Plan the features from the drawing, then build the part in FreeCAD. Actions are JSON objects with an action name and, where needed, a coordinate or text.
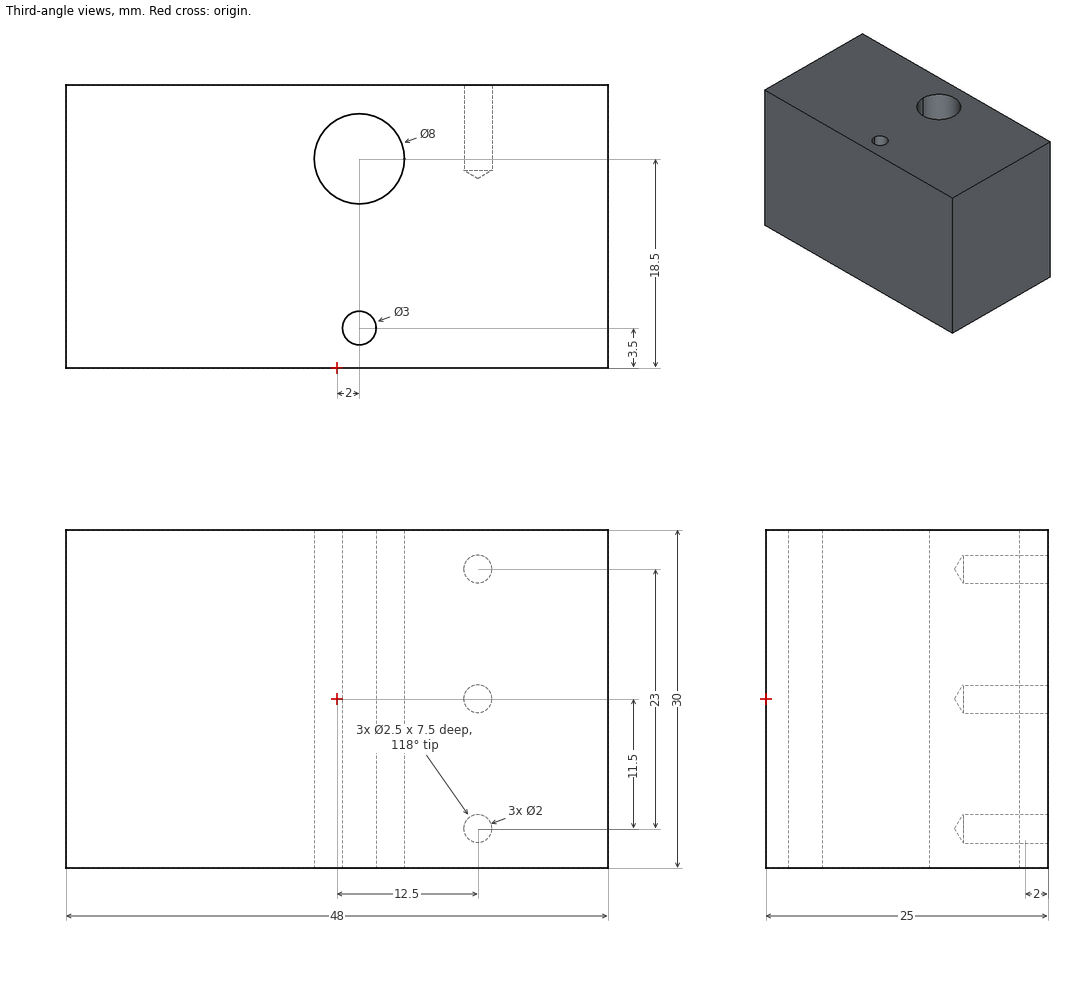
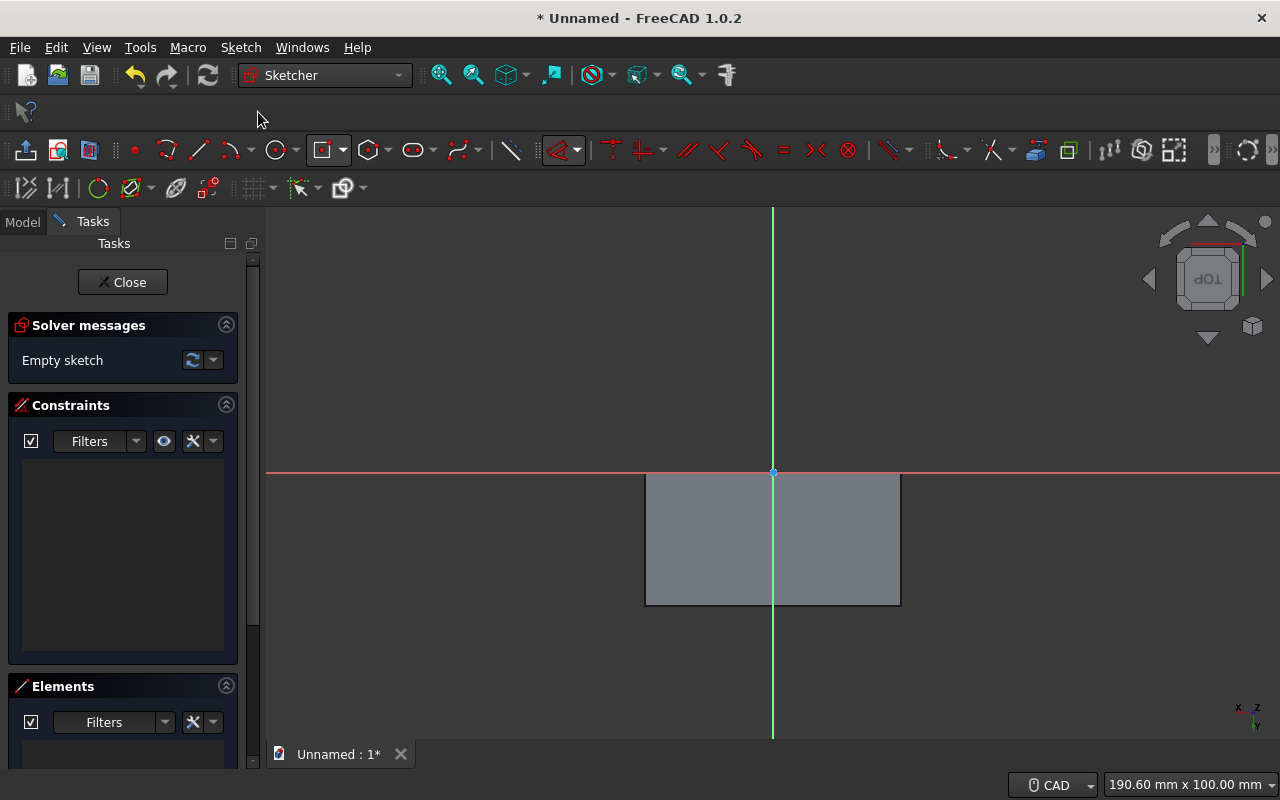
{"action": "scroll", "coordinate": [771, 587], "scroll_direction": "up", "scroll_amount": 10}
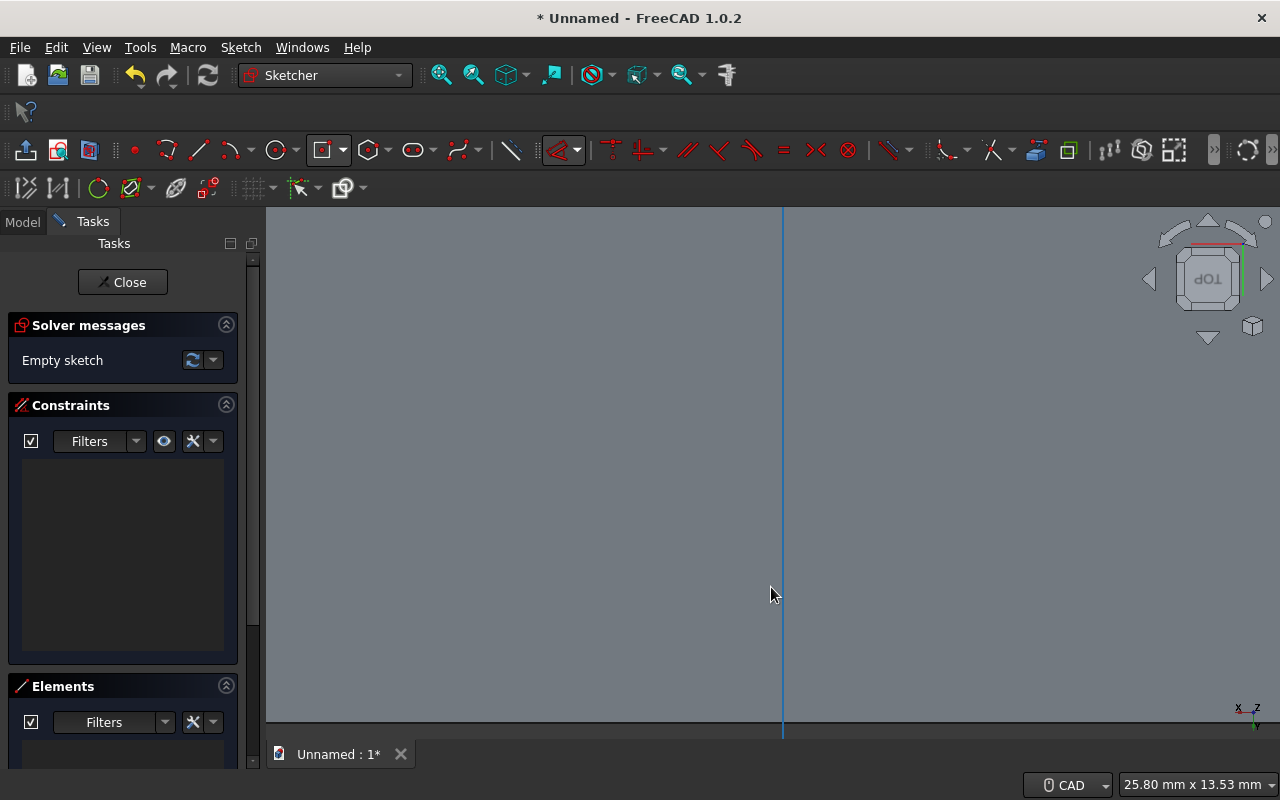
{"action": "left_click", "coordinate": [276, 150]}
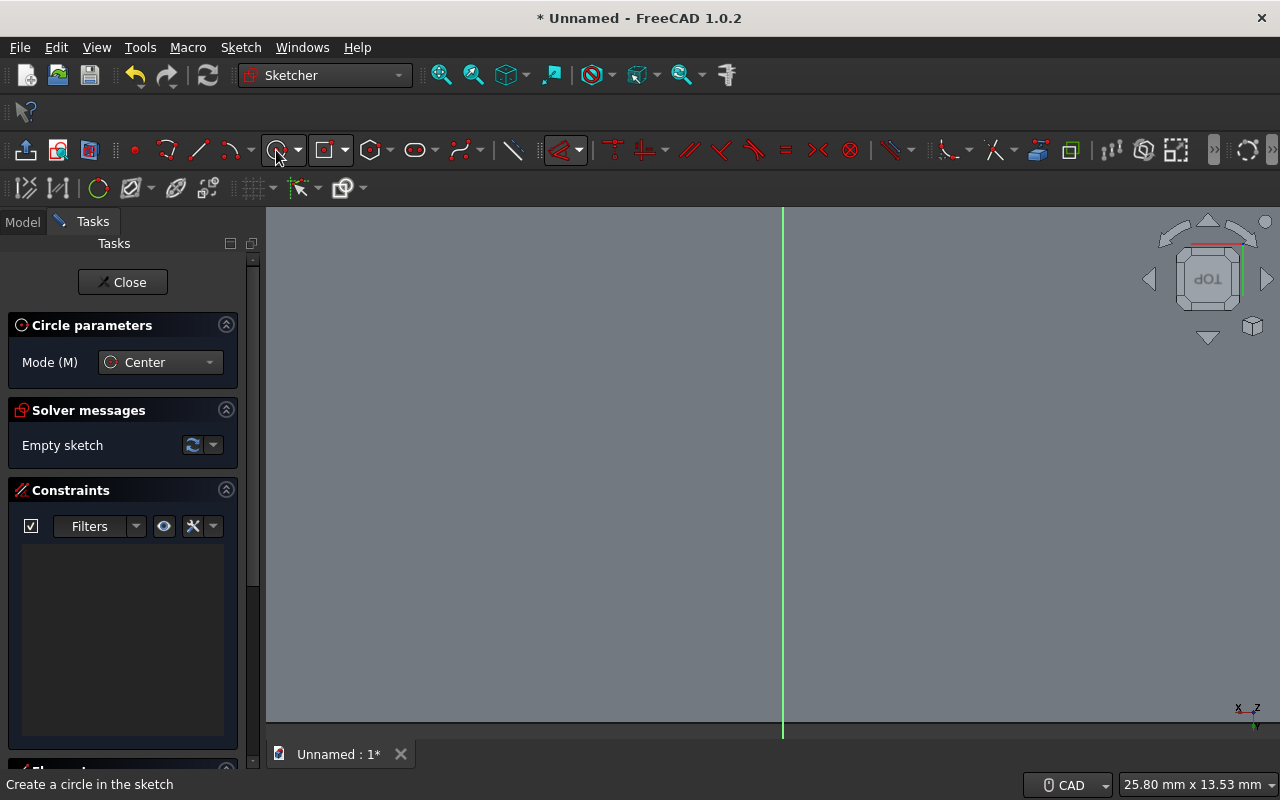
{"action": "left_click", "coordinate": [704, 467]}
{"action": "left_click", "coordinate": [815, 356]}
{"action": "key", "text": "Escape"}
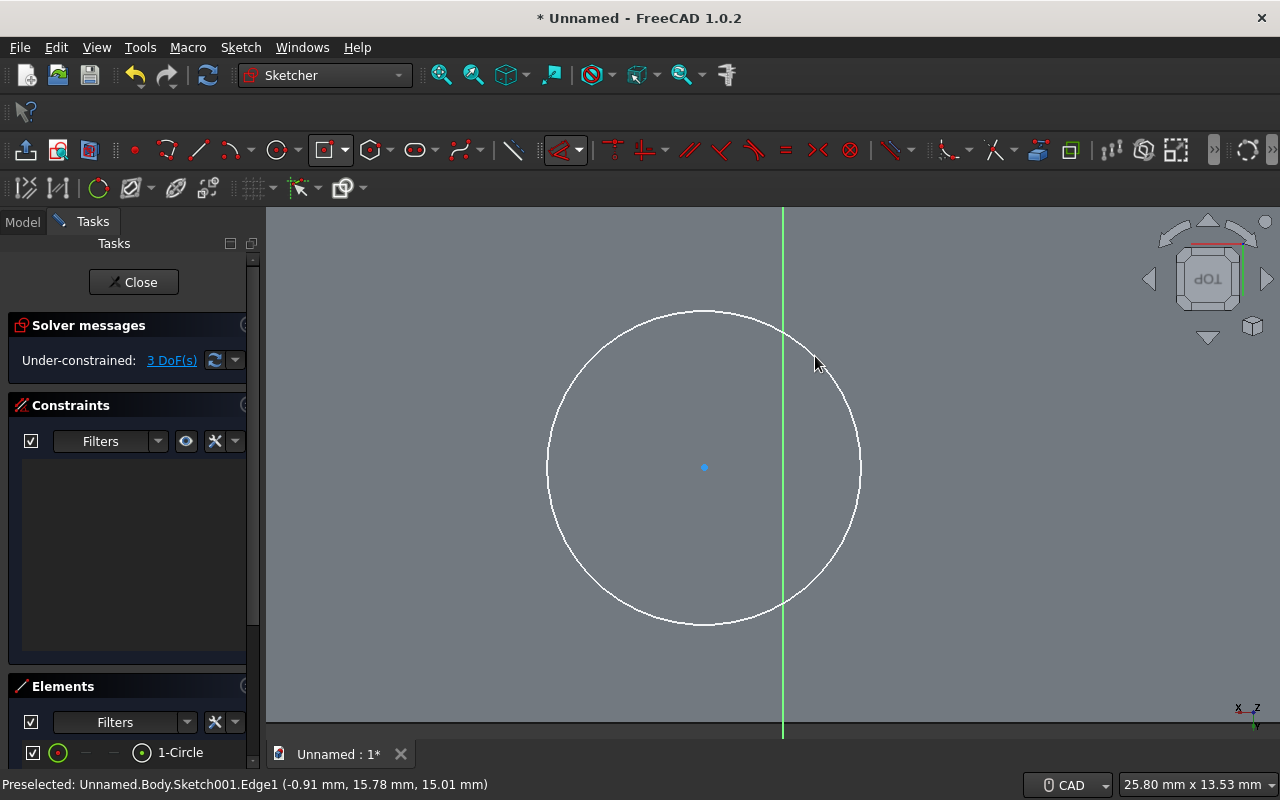
{"action": "left_click", "coordinate": [560, 150]}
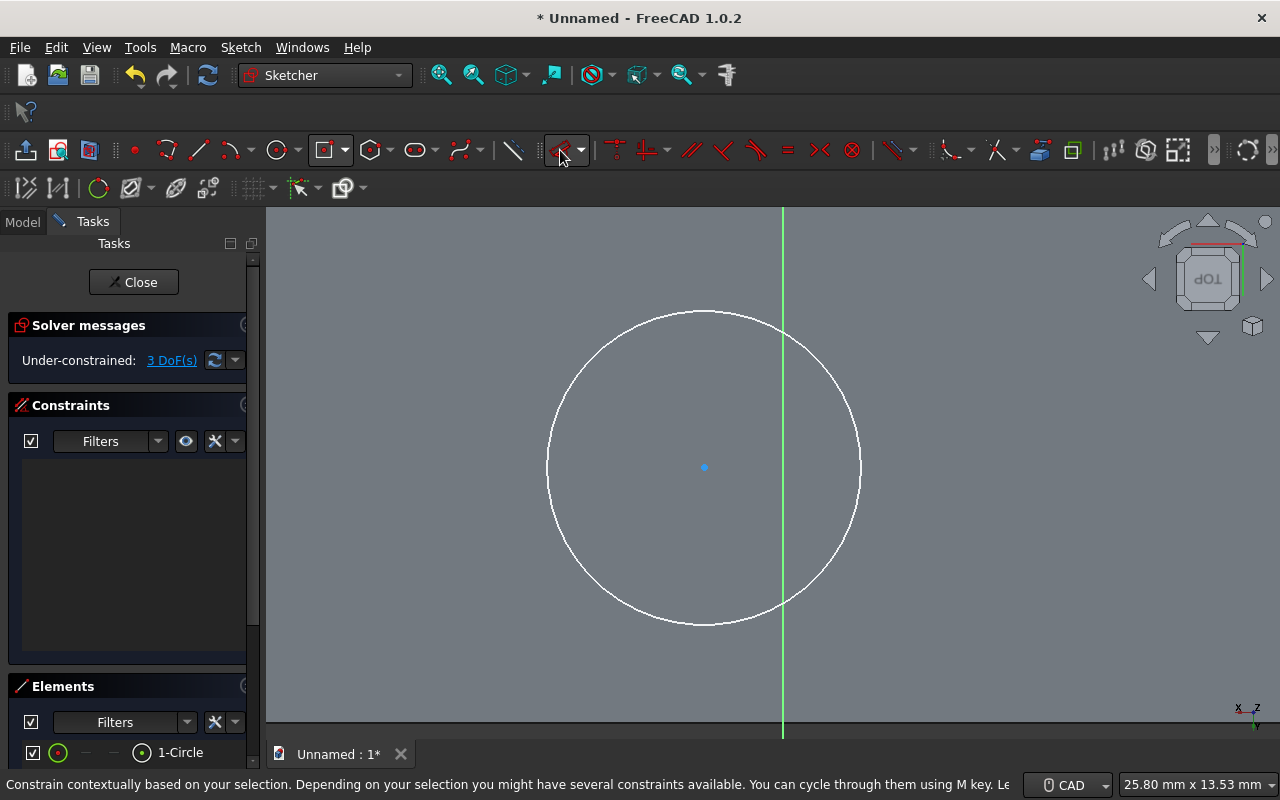
{"action": "left_click", "coordinate": [815, 357]}
{"action": "left_click", "coordinate": [838, 334]}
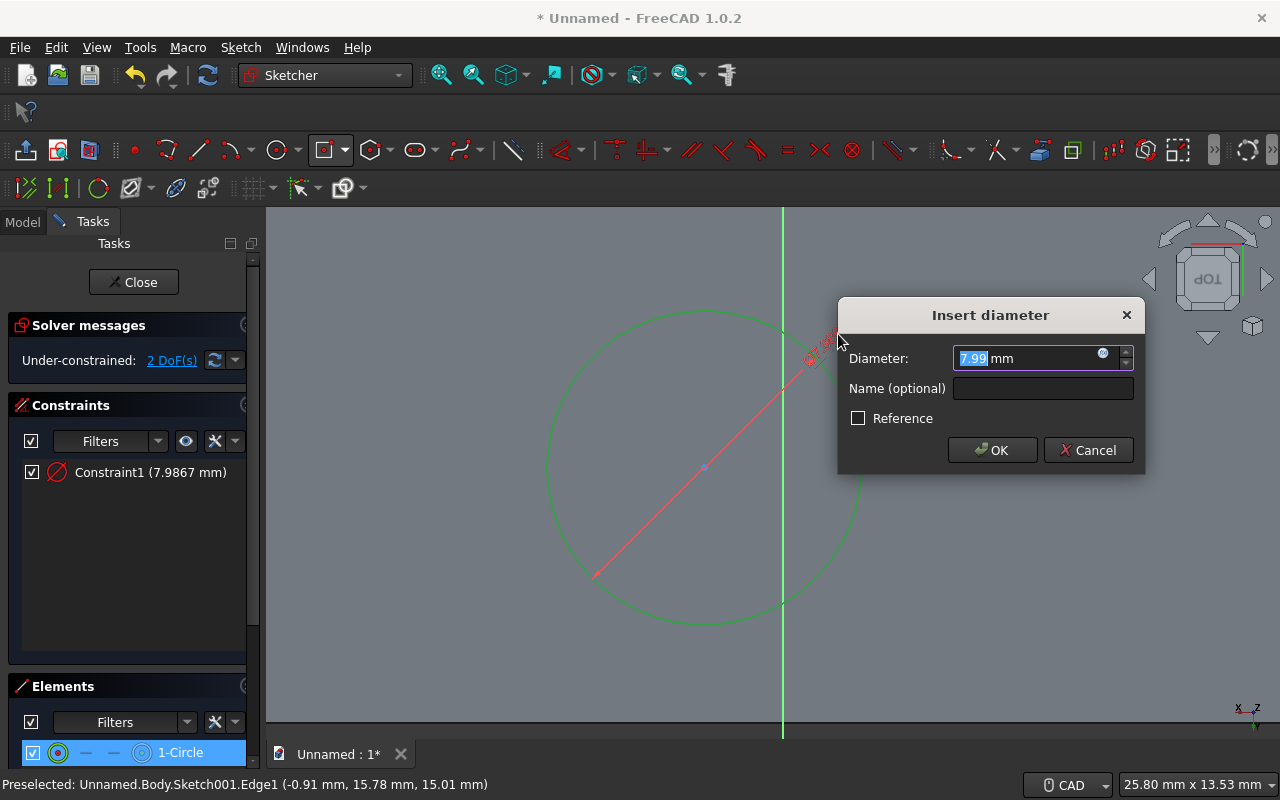
{"action": "type", "text": "8"}
{"action": "key", "text": "Return"}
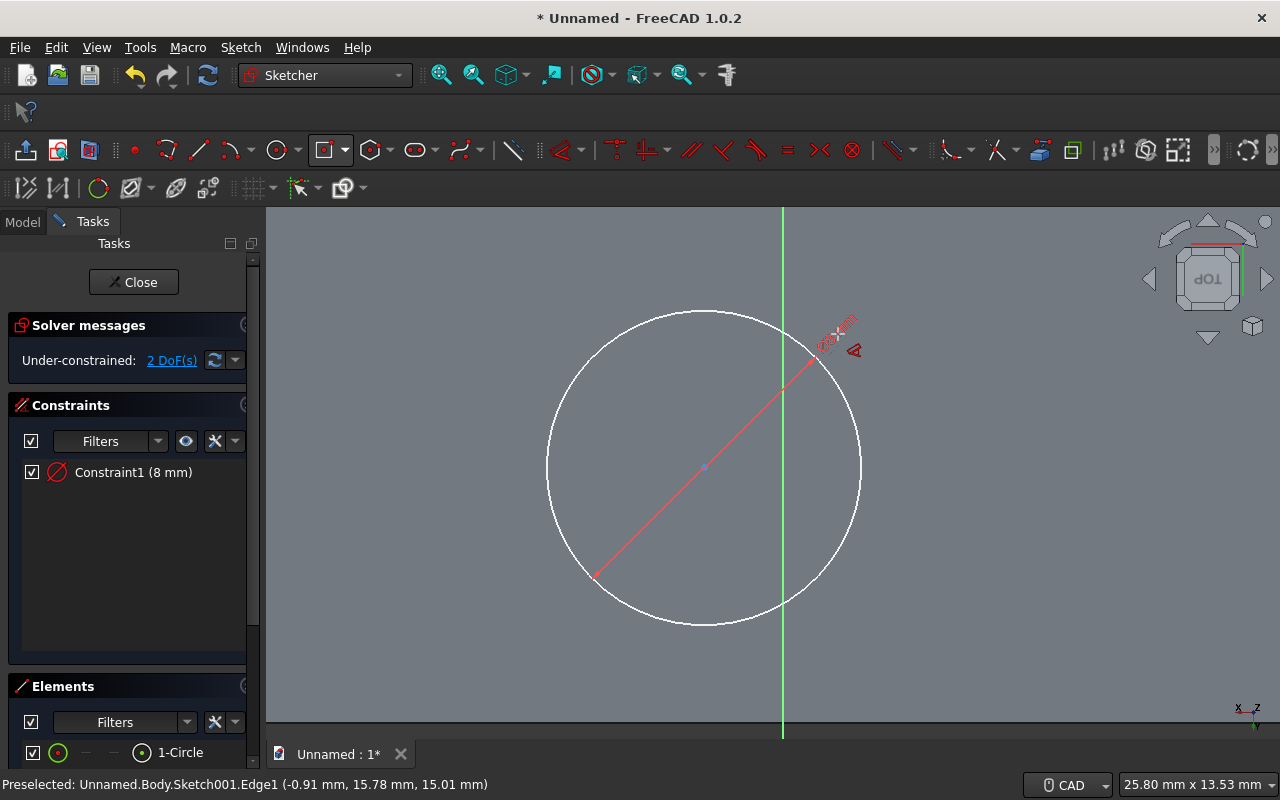
{"action": "left_click", "coordinate": [704, 468]}
{"action": "left_click", "coordinate": [743, 502]}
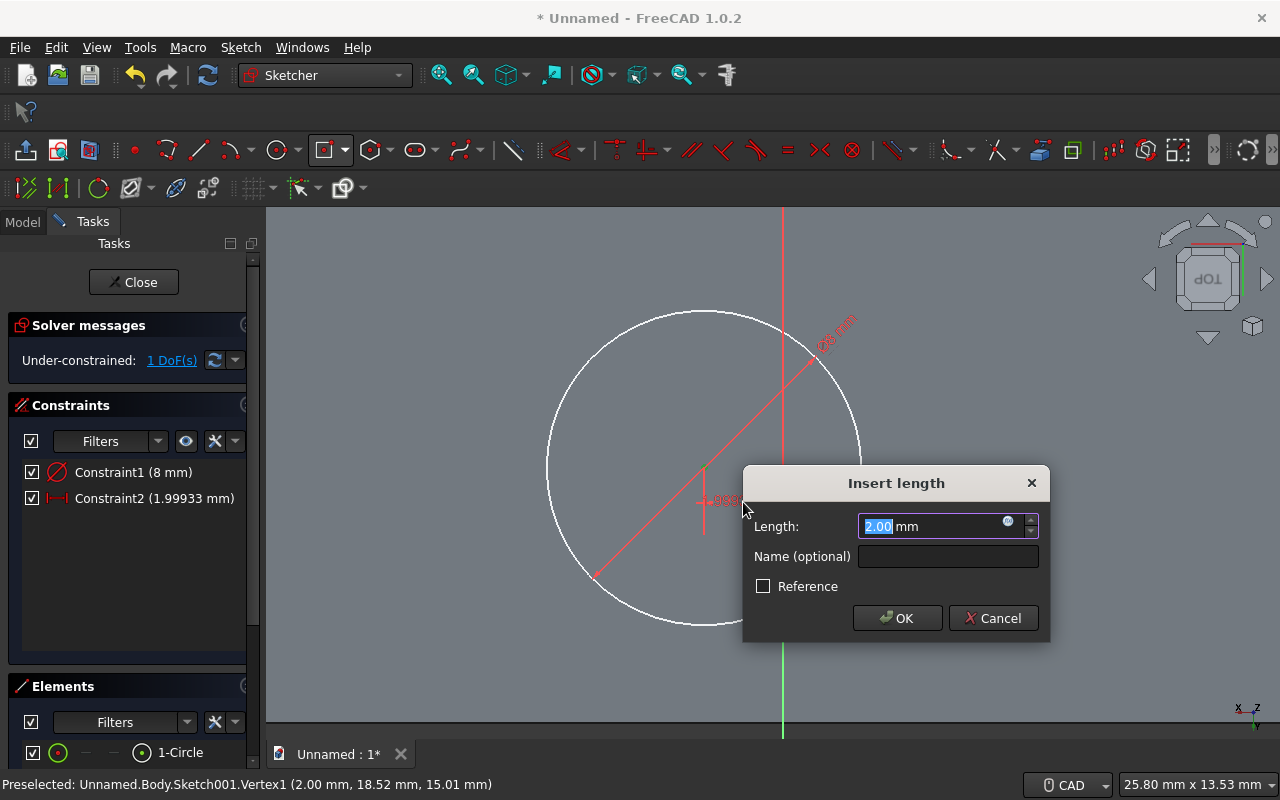
{"action": "type", "text": "2"}
{"action": "key", "text": "Return"}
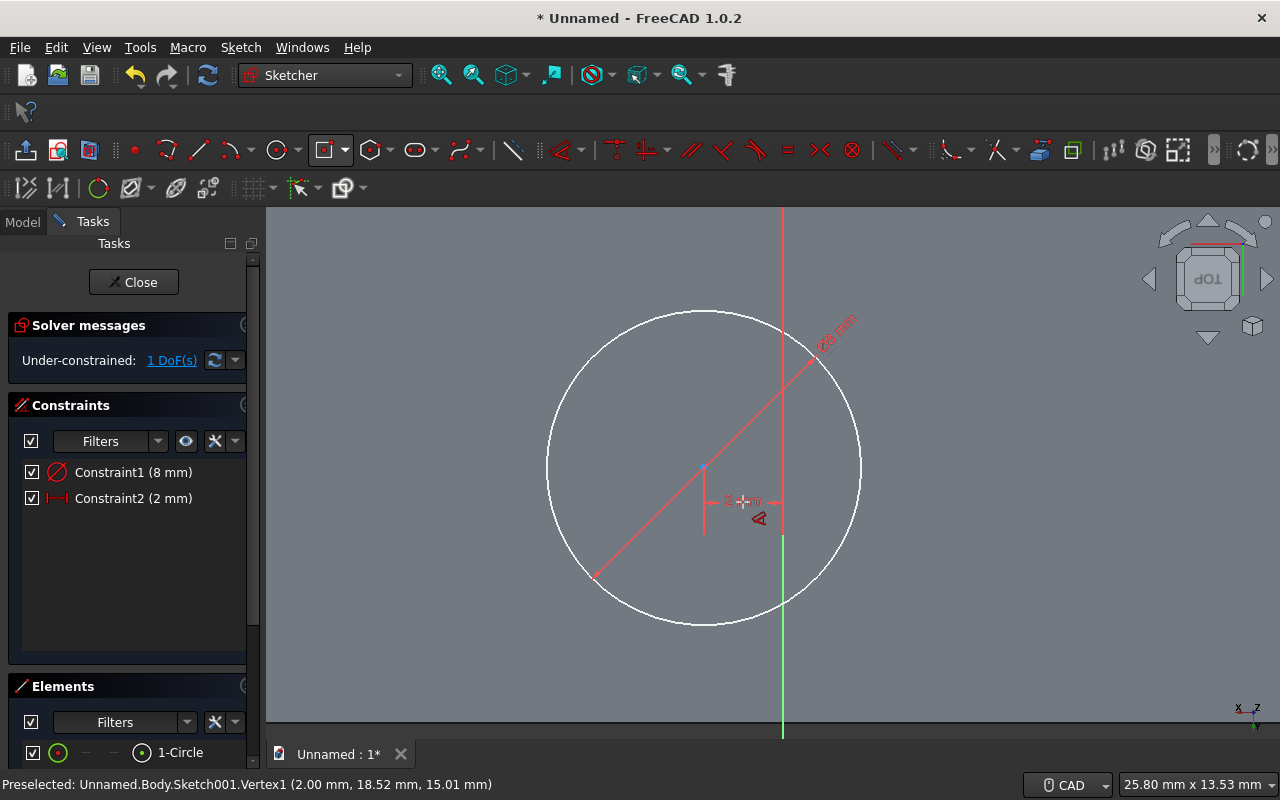
{"action": "left_click", "coordinate": [704, 468]}
{"action": "left_click", "coordinate": [817, 298]}